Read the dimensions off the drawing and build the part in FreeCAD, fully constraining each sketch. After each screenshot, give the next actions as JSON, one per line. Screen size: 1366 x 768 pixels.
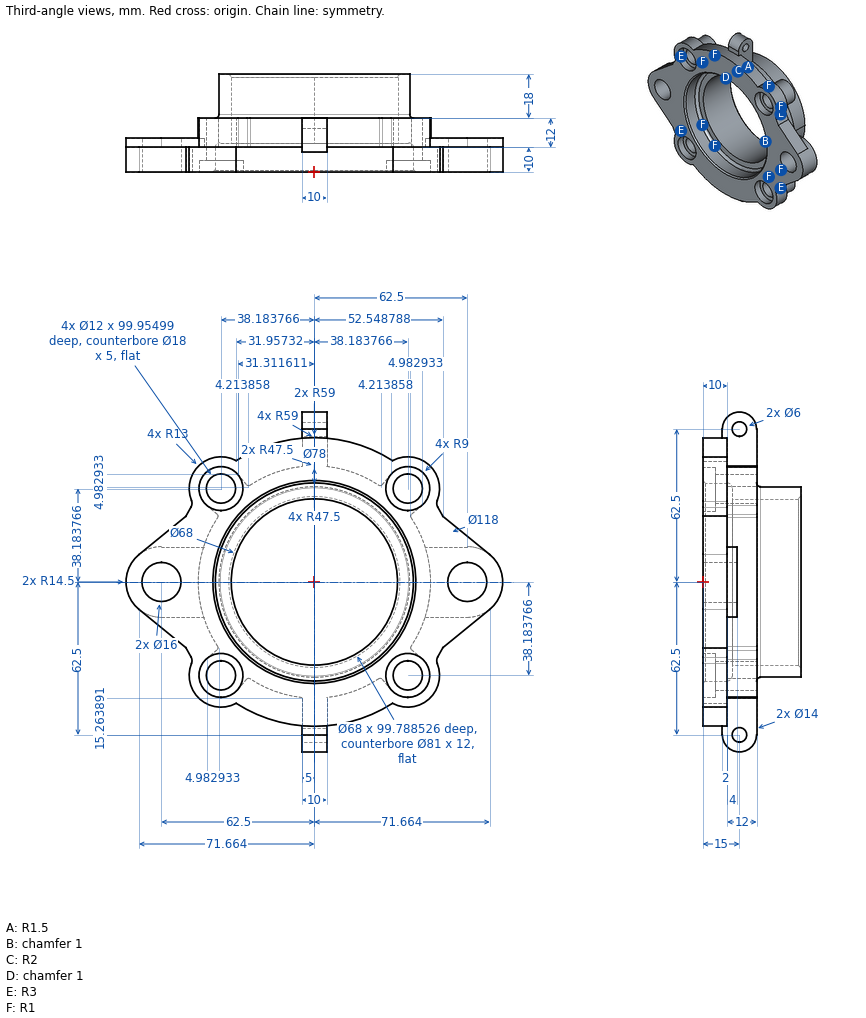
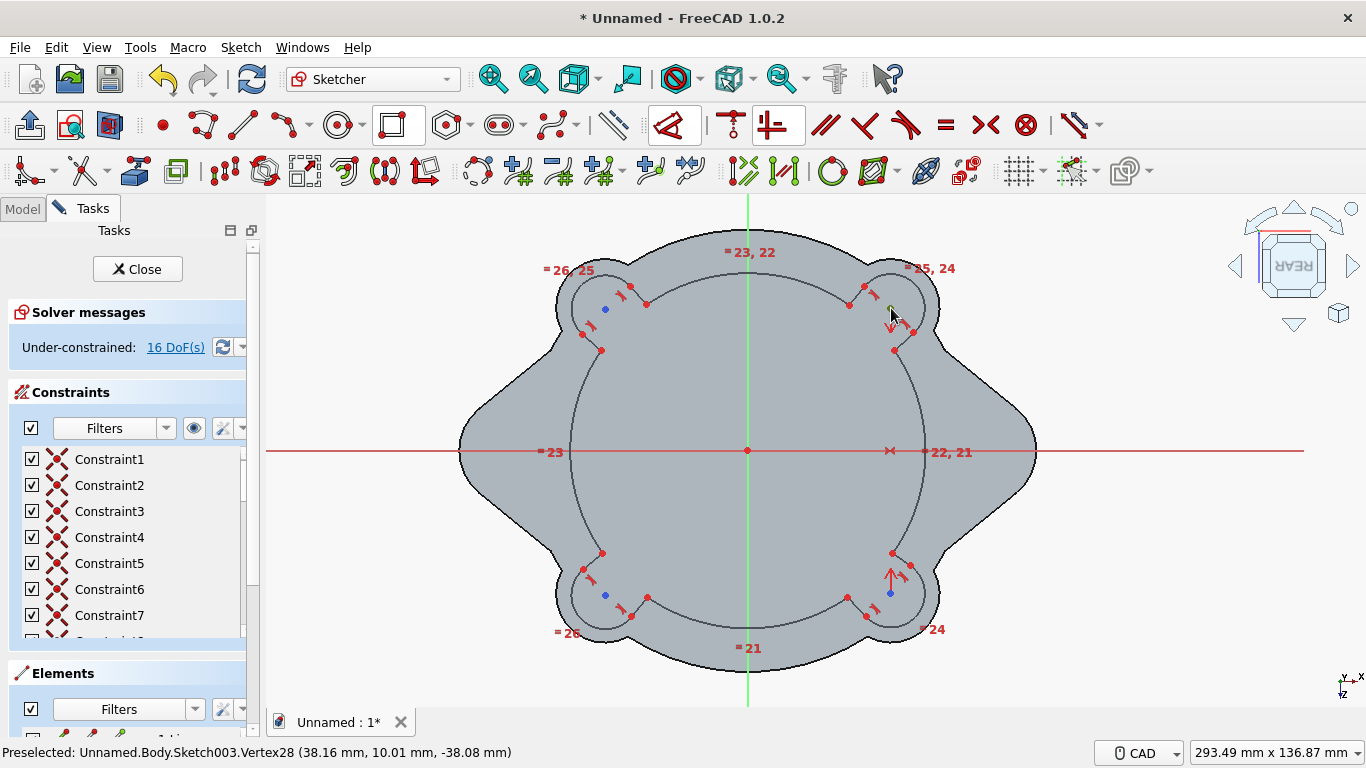
{"action": "left_click", "coordinate": [605, 309]}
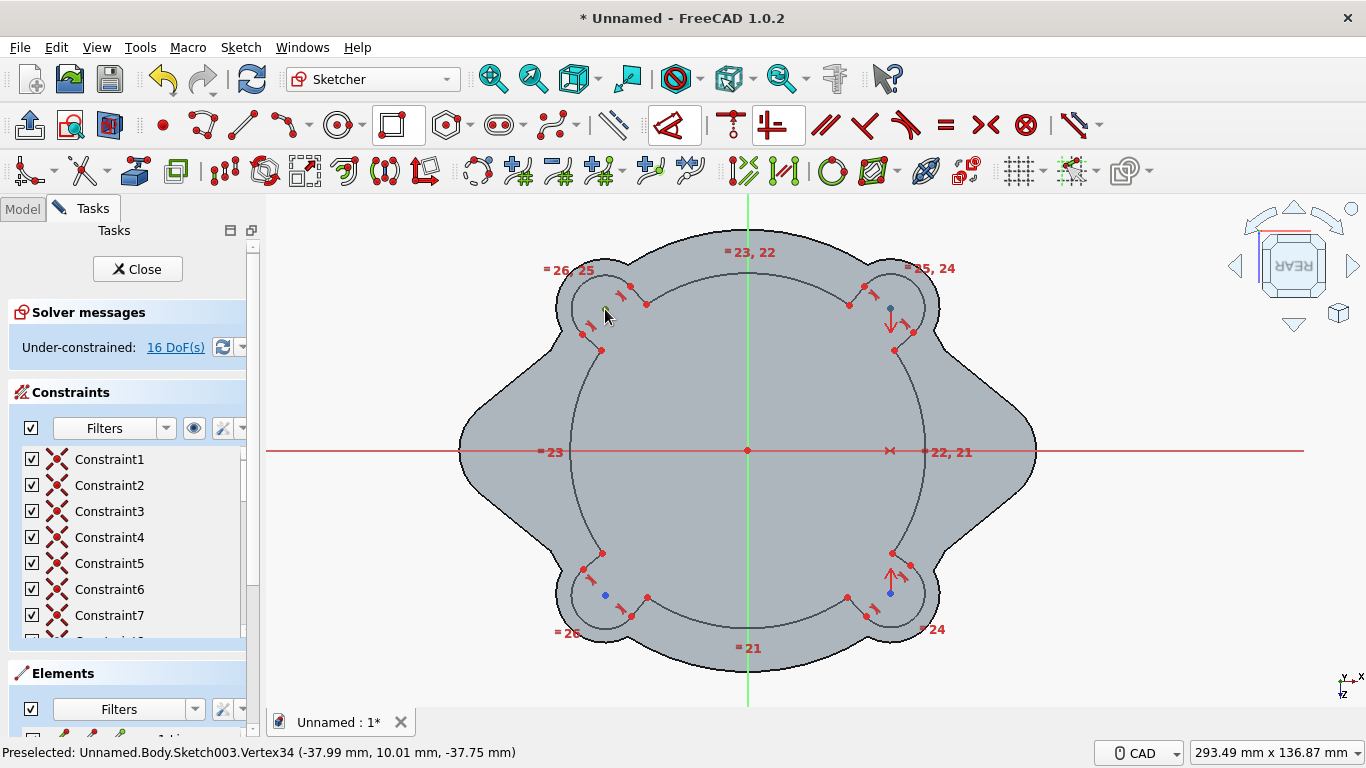
{"action": "left_click", "coordinate": [748, 581]}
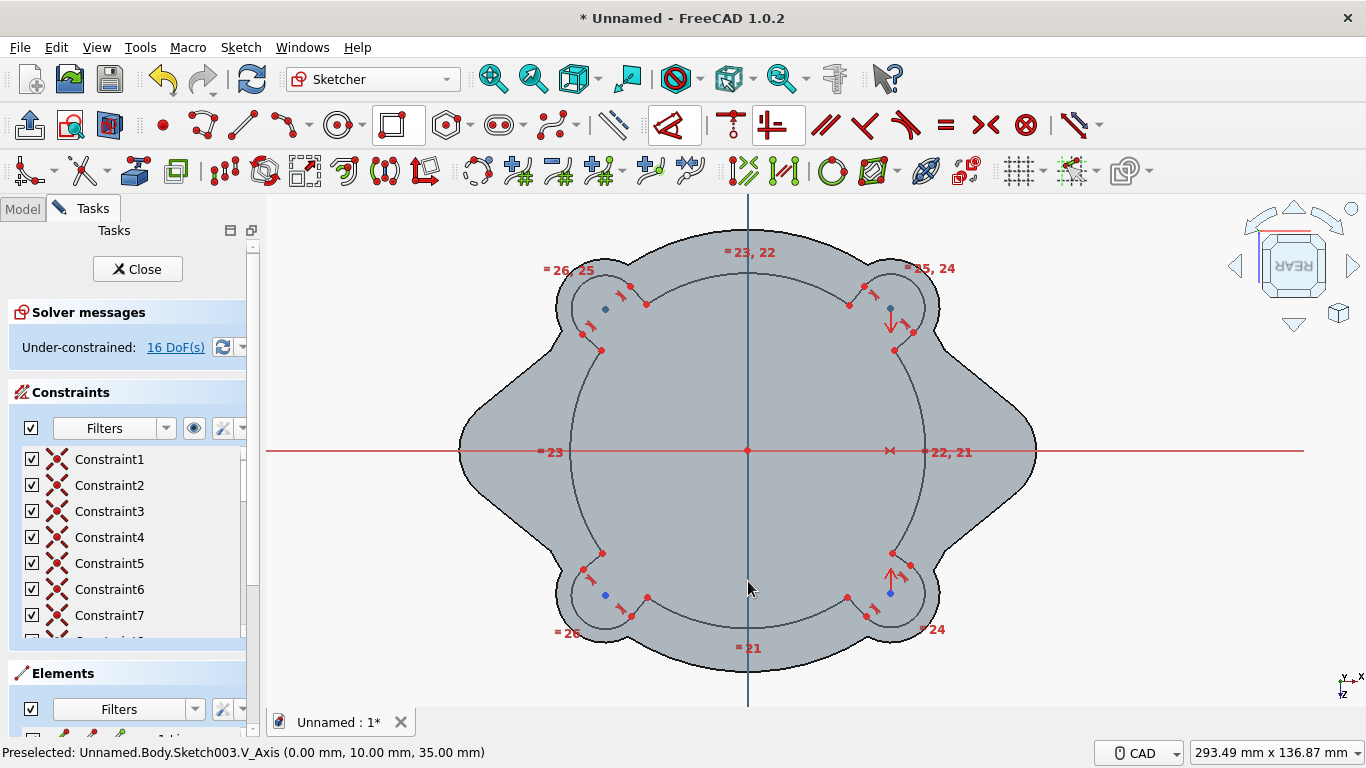
{"action": "left_click", "coordinate": [986, 126]}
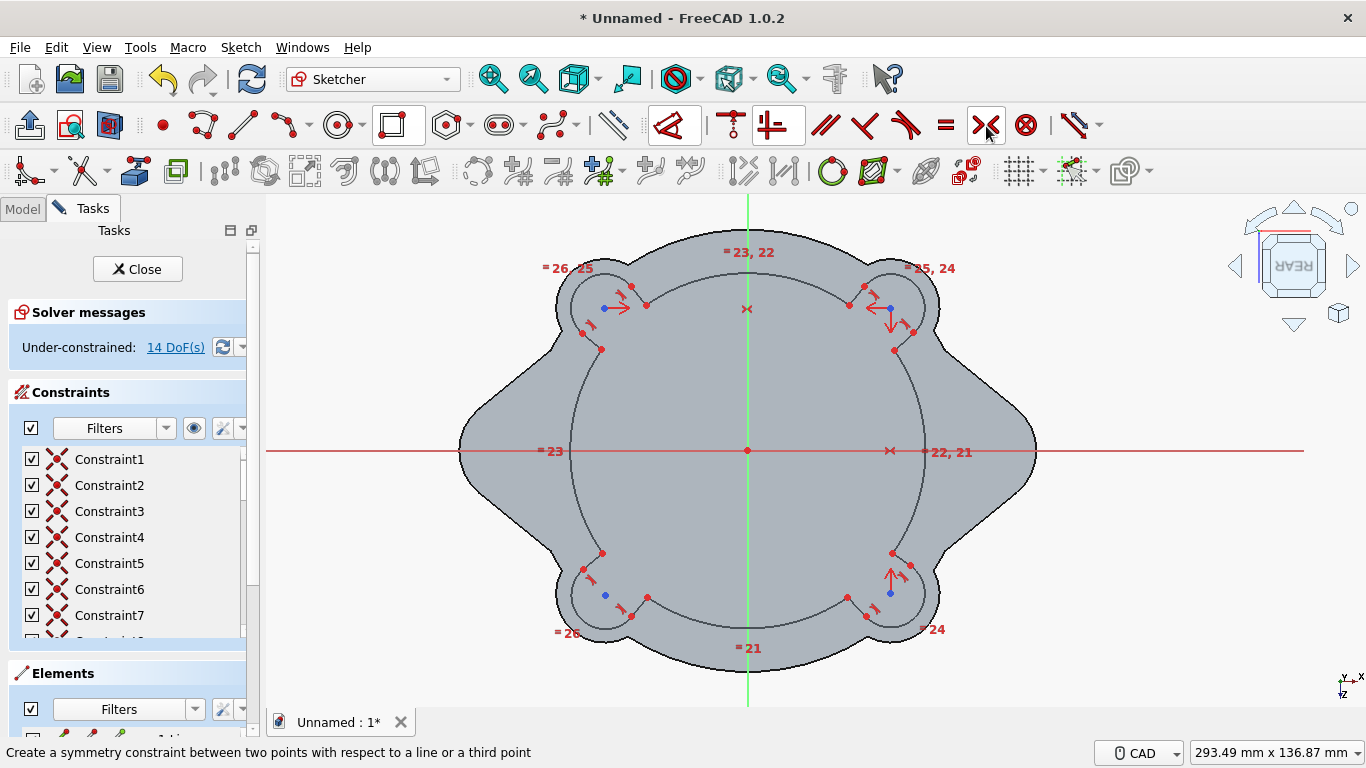
{"action": "left_click", "coordinate": [891, 594]}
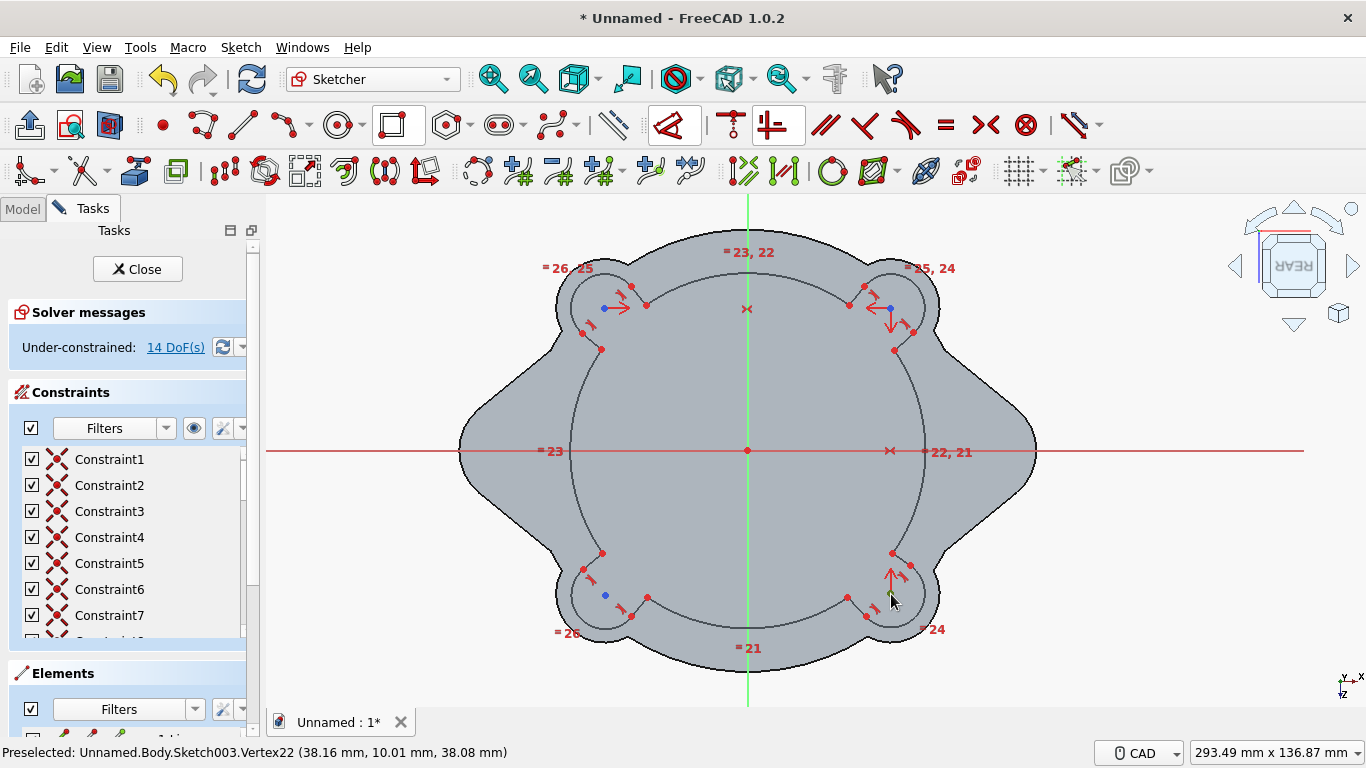
{"action": "left_click", "coordinate": [605, 595]}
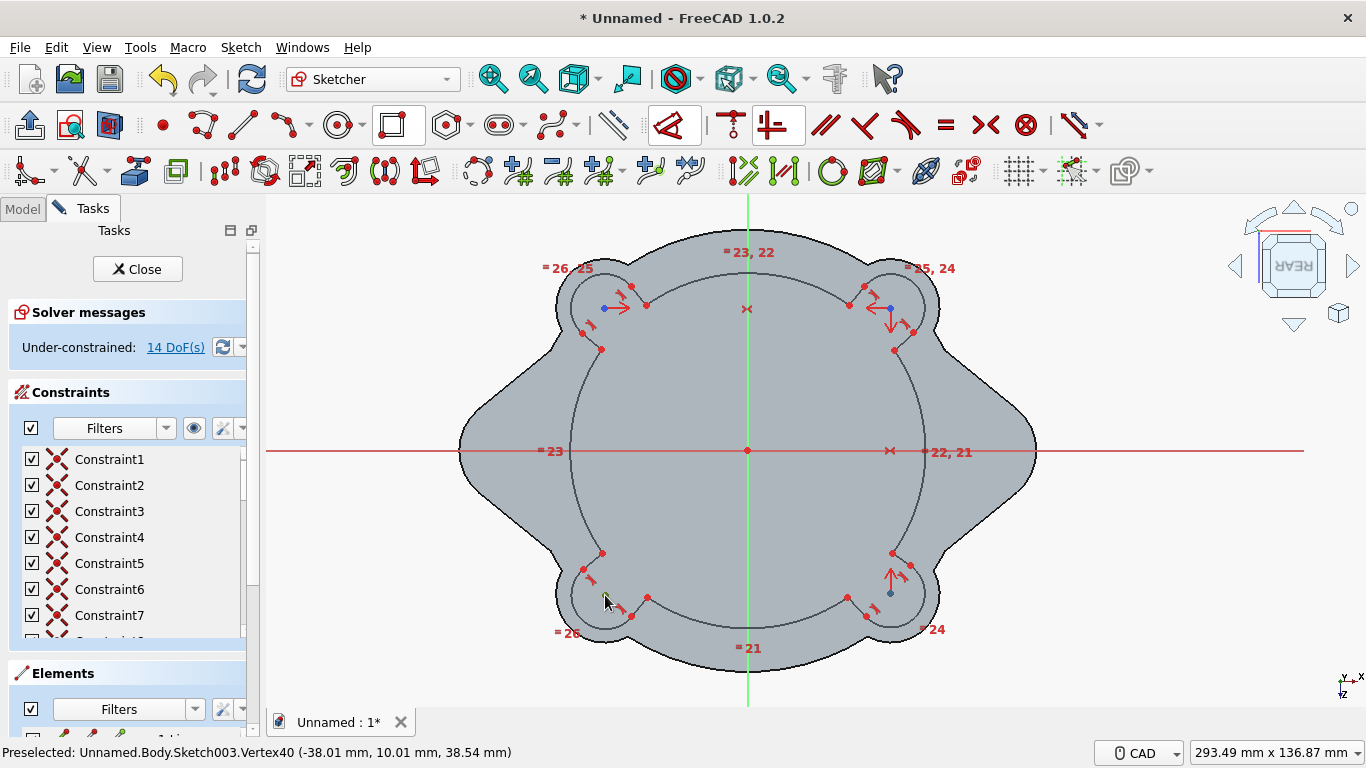
{"action": "left_click", "coordinate": [748, 581]}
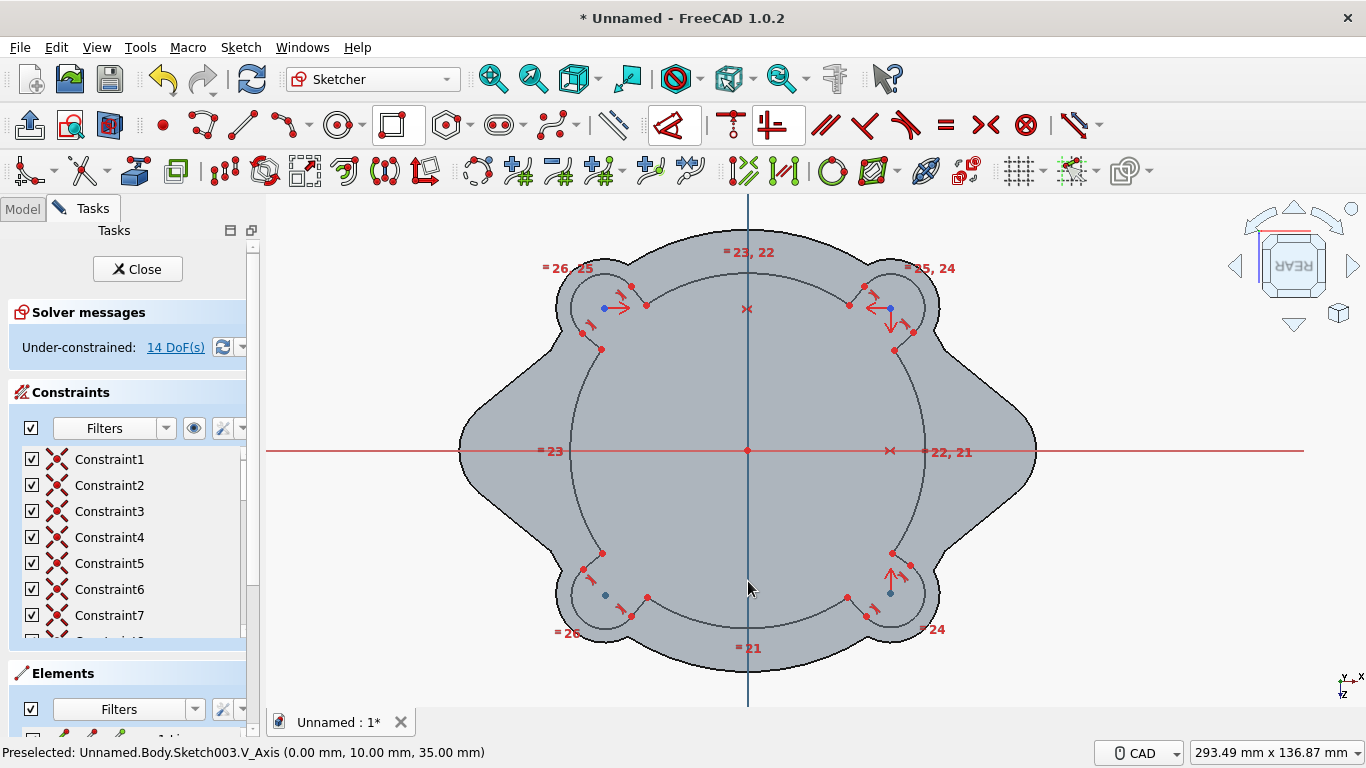
{"action": "left_click", "coordinate": [986, 126]}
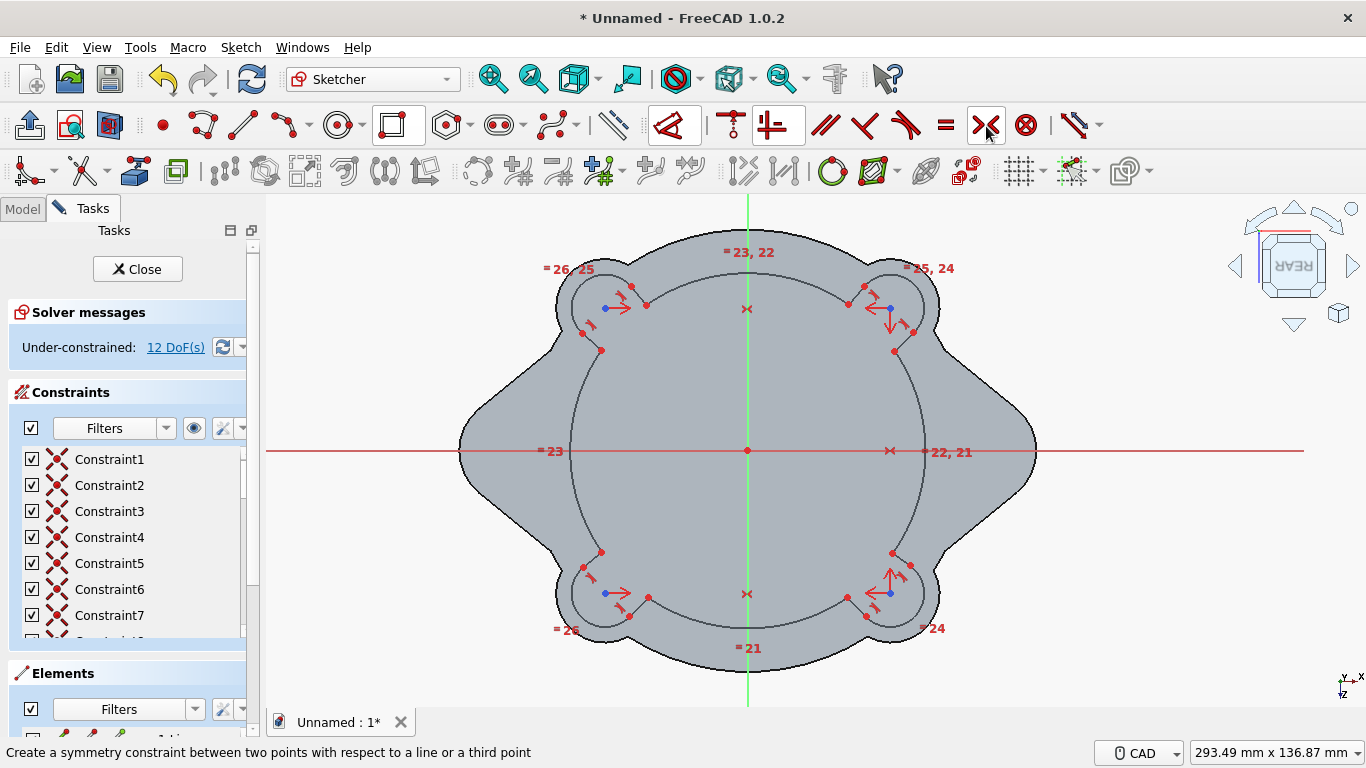
{"action": "left_click", "coordinate": [706, 623]}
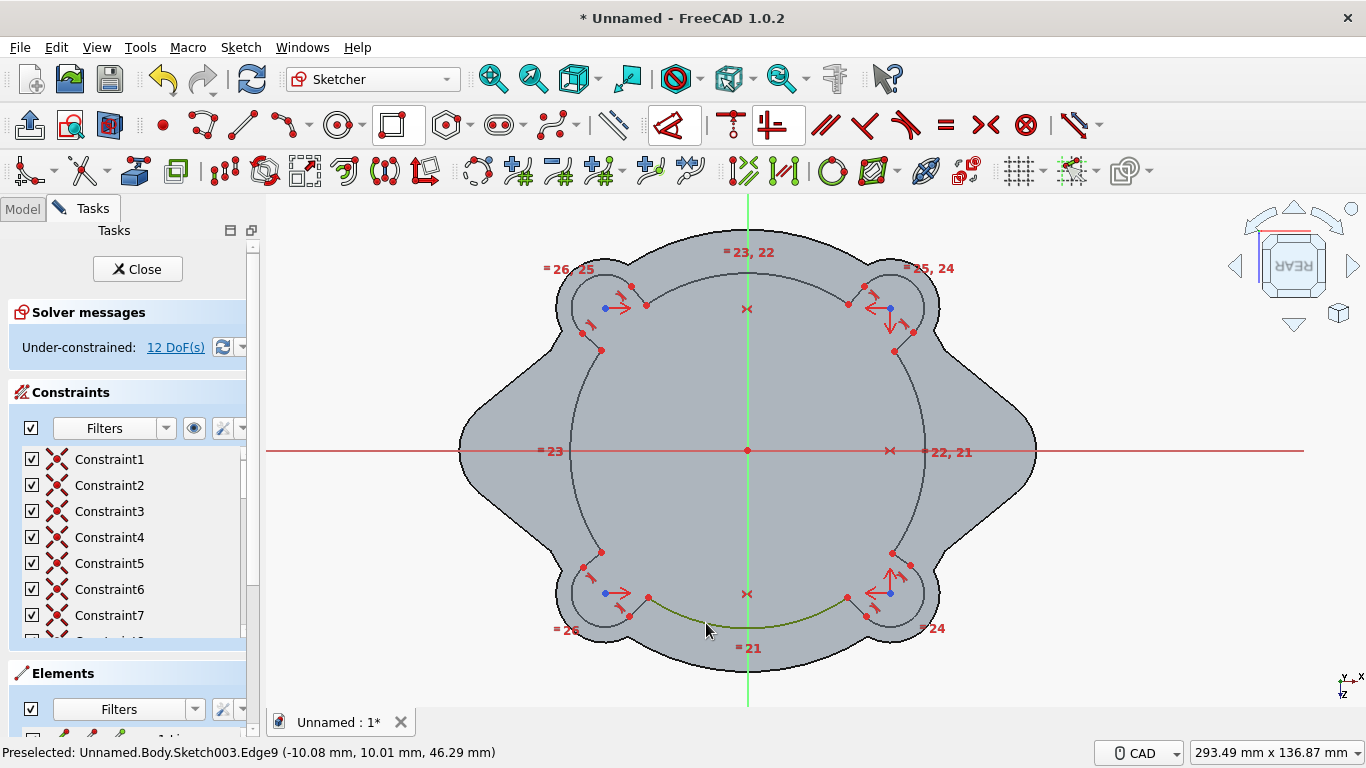
{"action": "key", "text": "k r"}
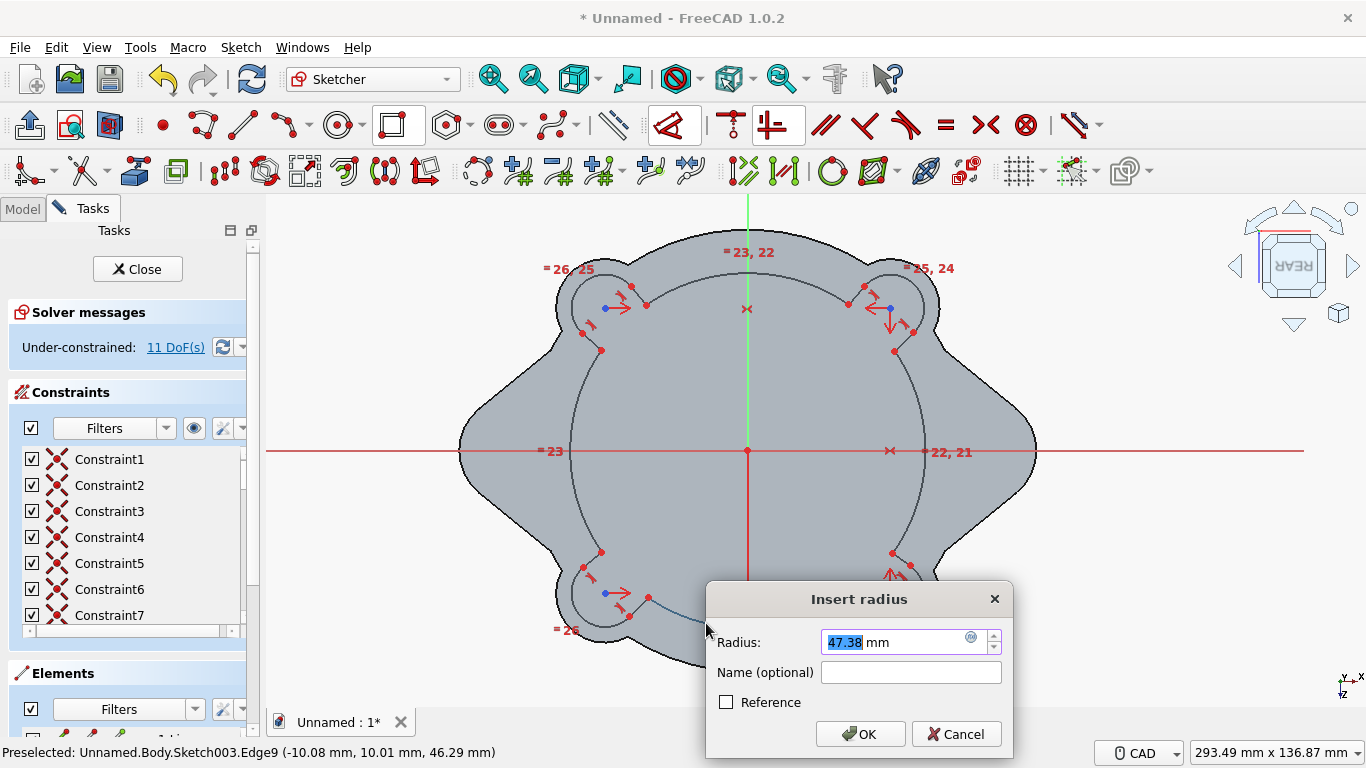
{"action": "type", "text": "47.5"}
{"action": "key", "text": "Return"}